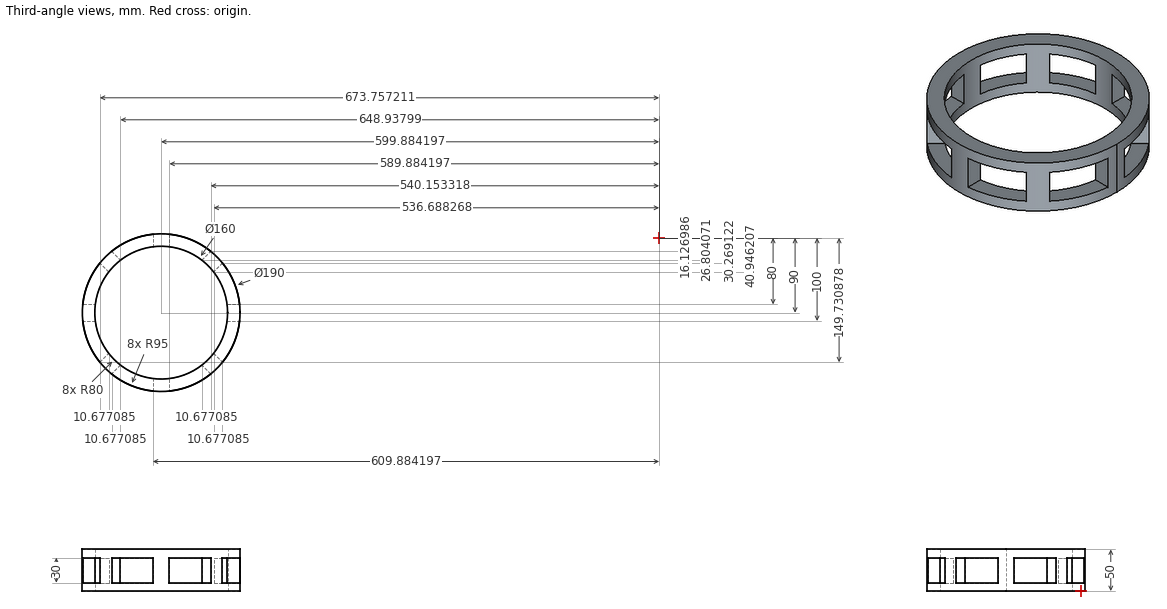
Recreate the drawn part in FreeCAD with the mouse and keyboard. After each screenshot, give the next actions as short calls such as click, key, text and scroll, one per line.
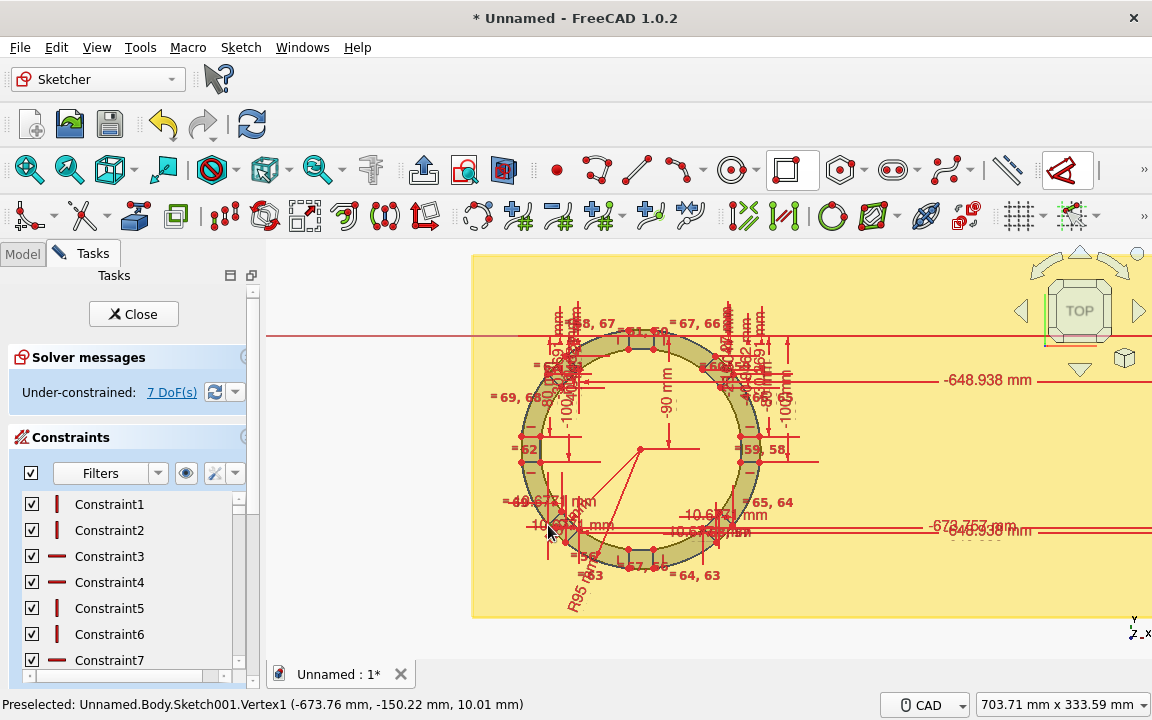
key(i)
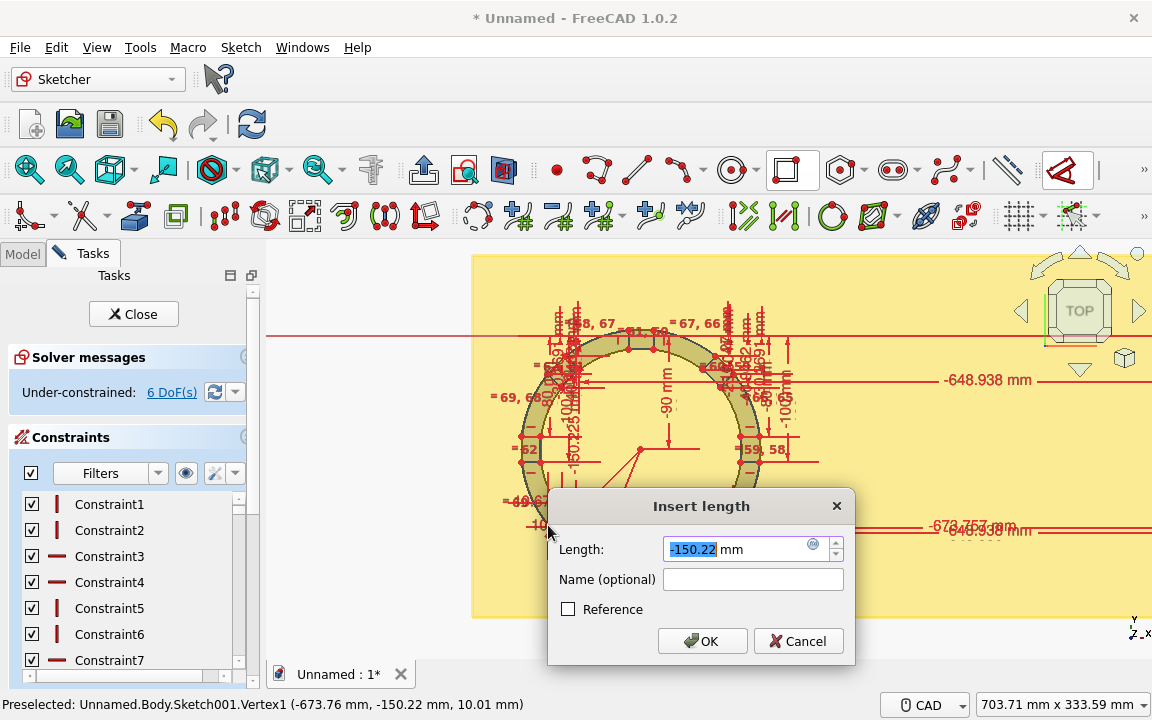
text(-149.730878)
key(Return)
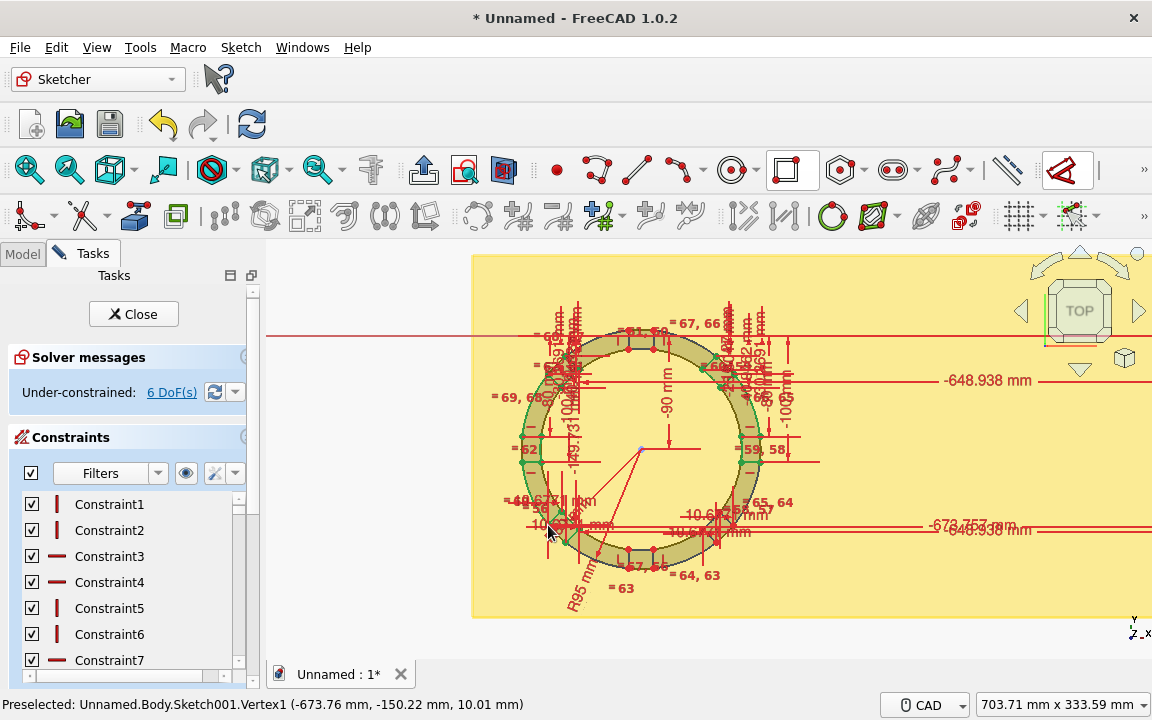
click(629, 568)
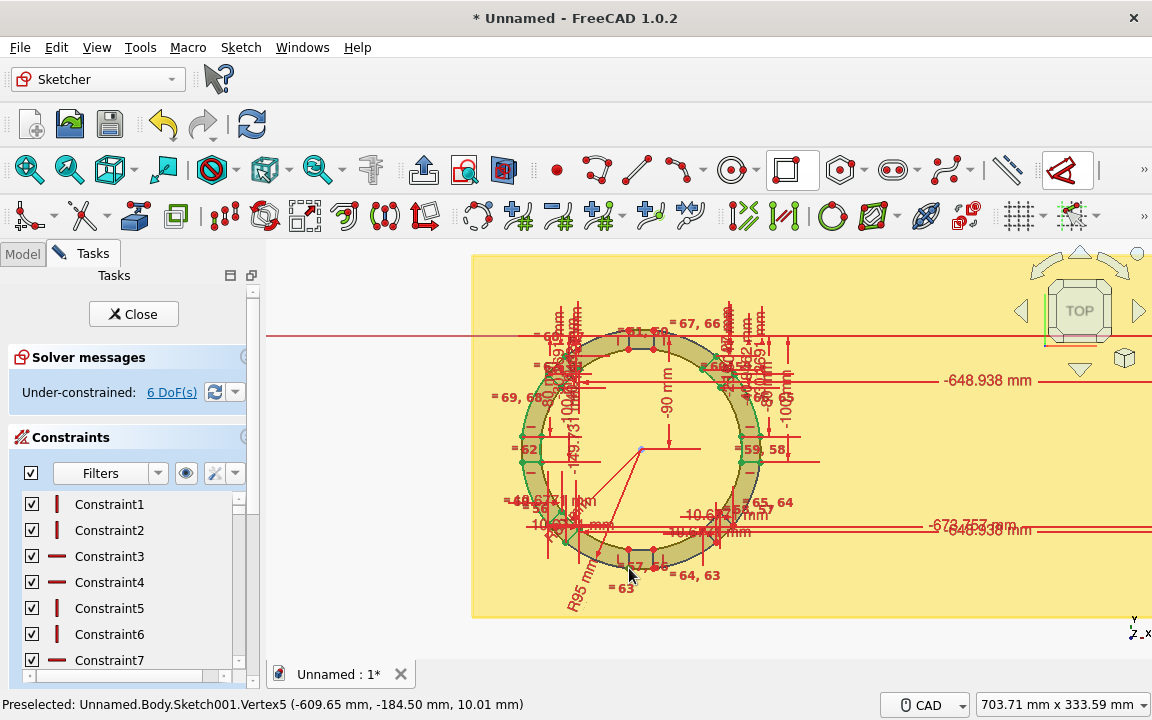
click(1088, 170)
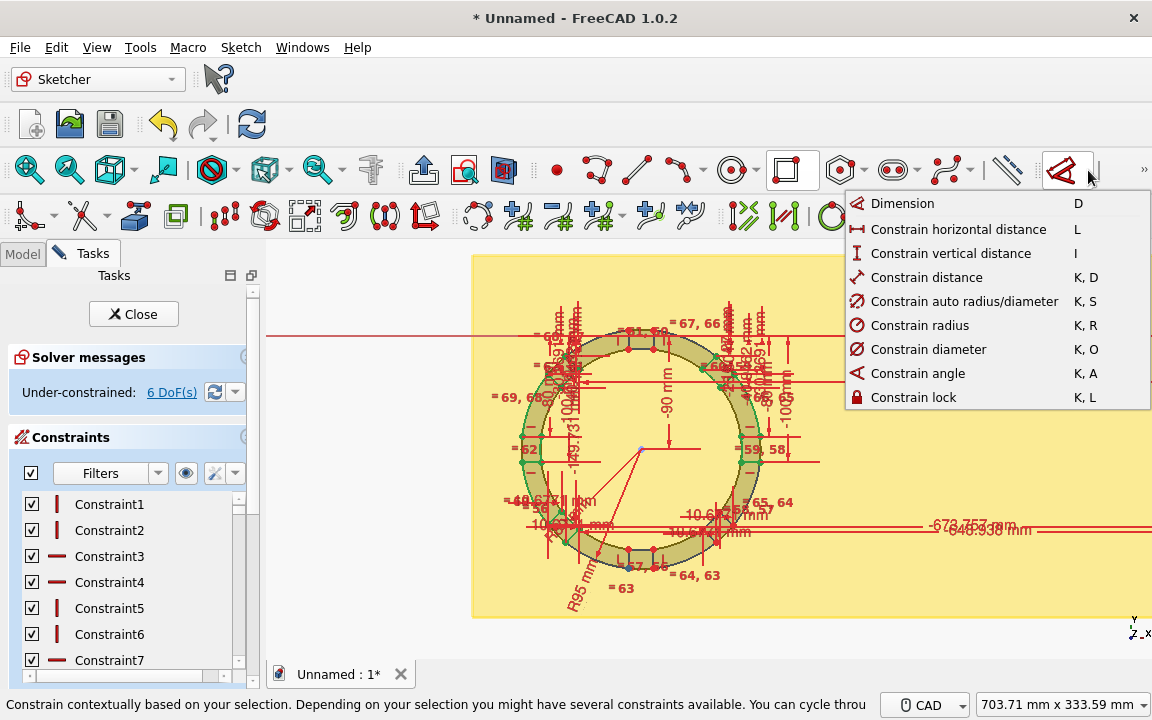
click(998, 229)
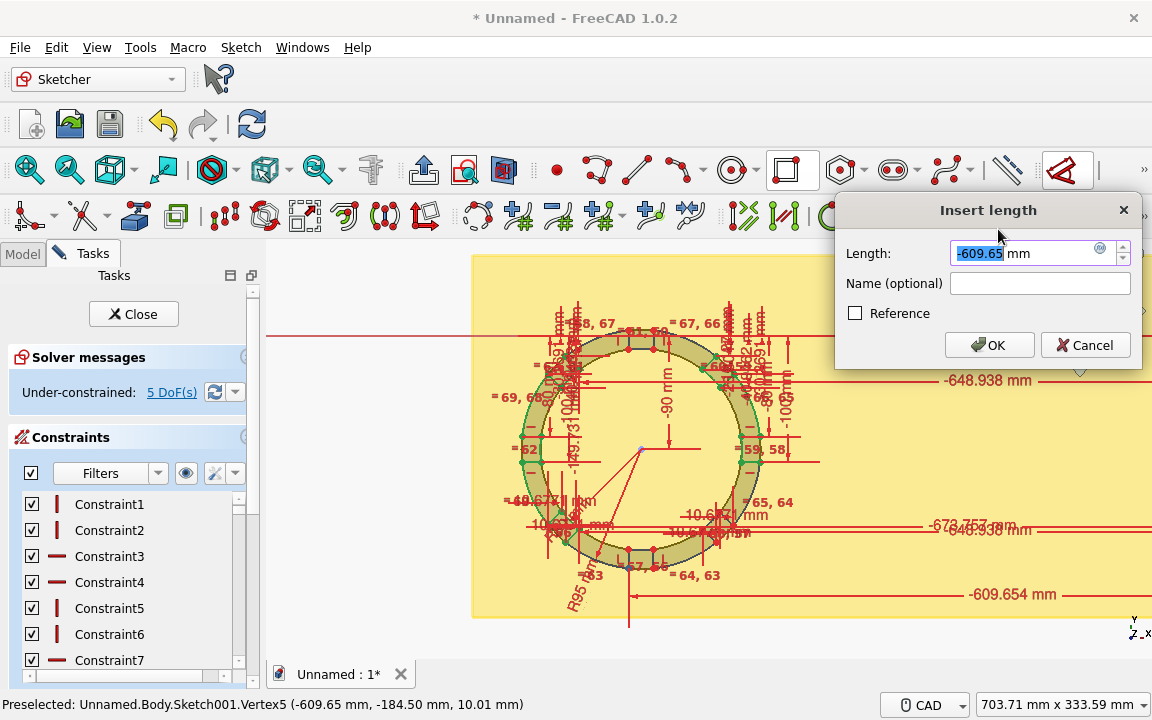
text(-609.884197)
key(Return)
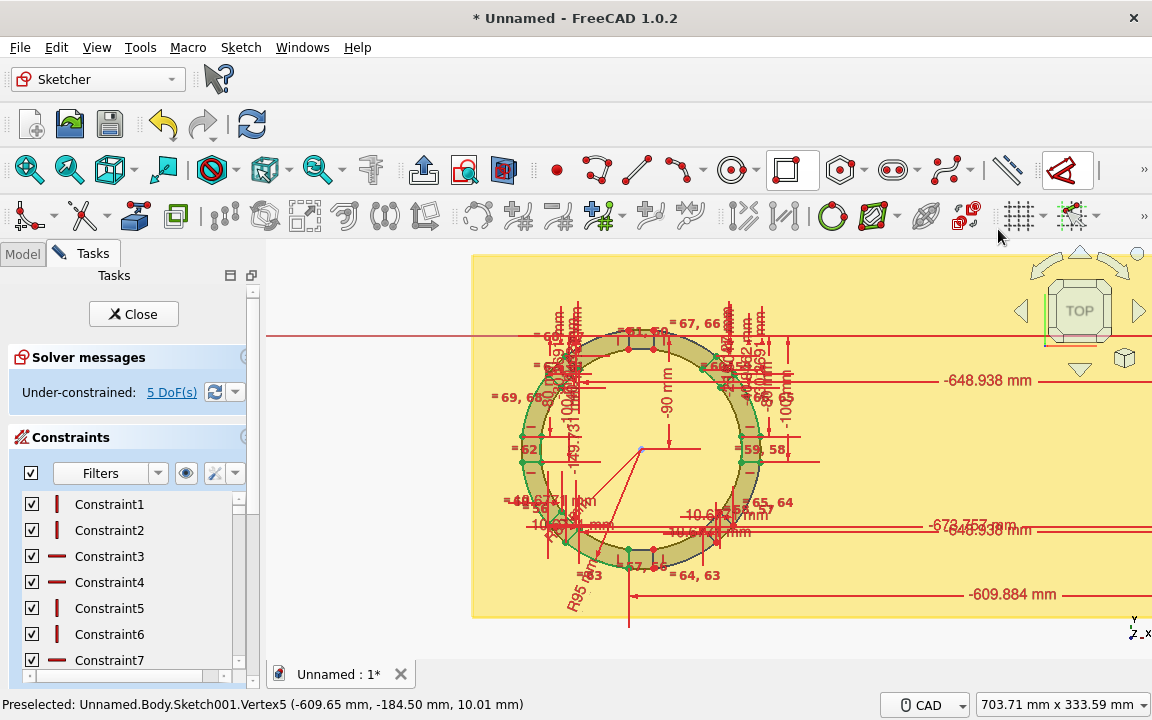
click(653, 549)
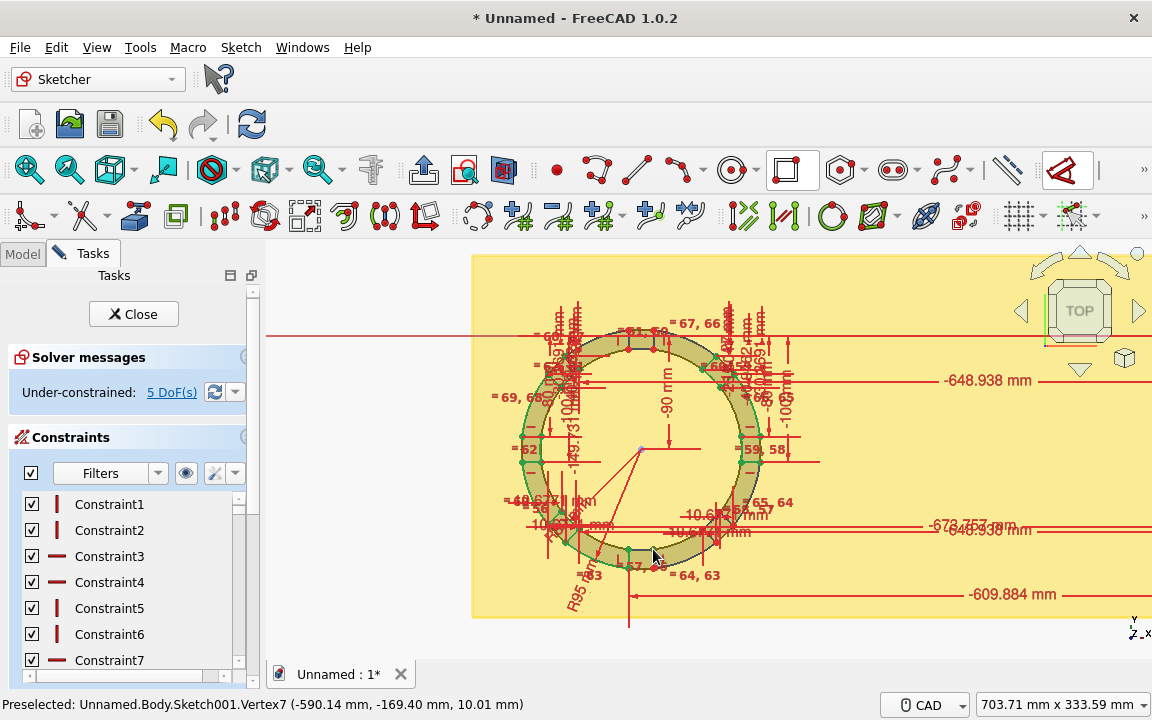
key(l)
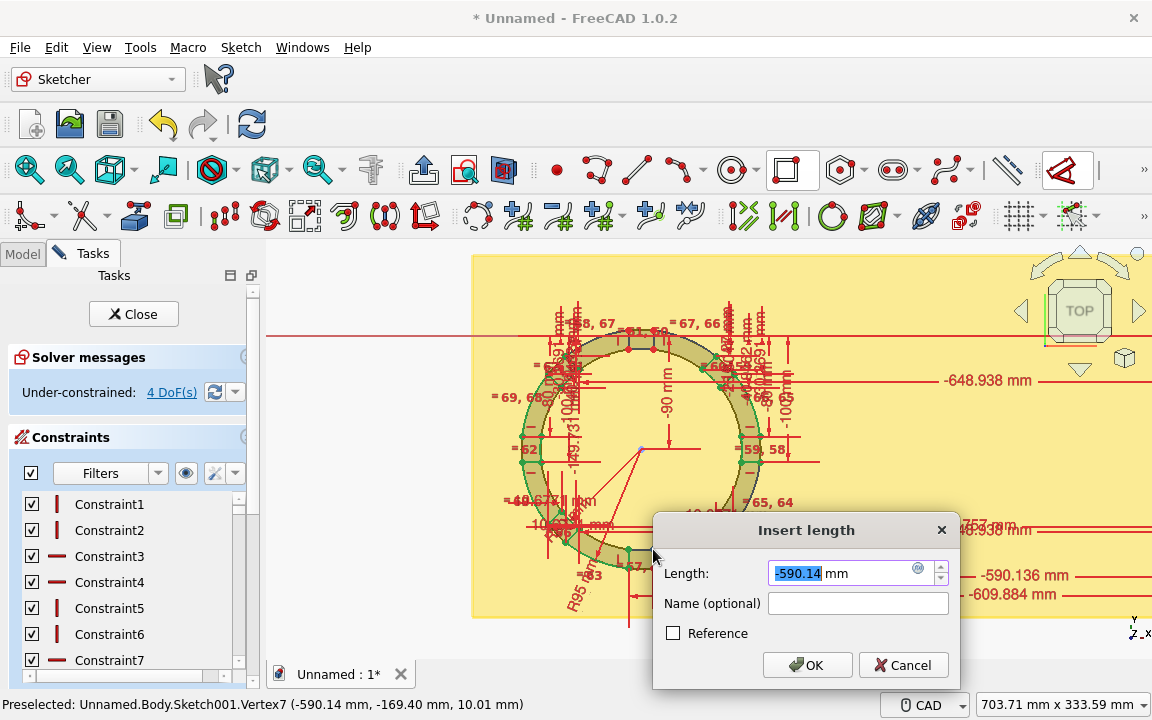
text(-589.884197)
key(Return)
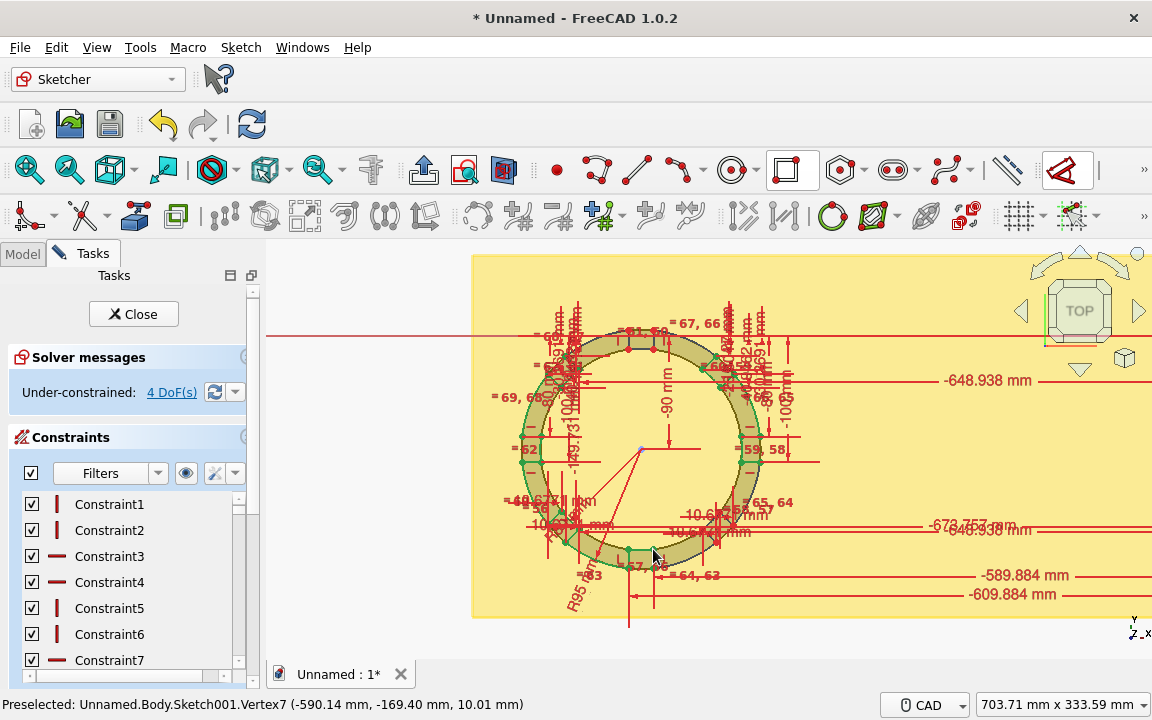
click(716, 542)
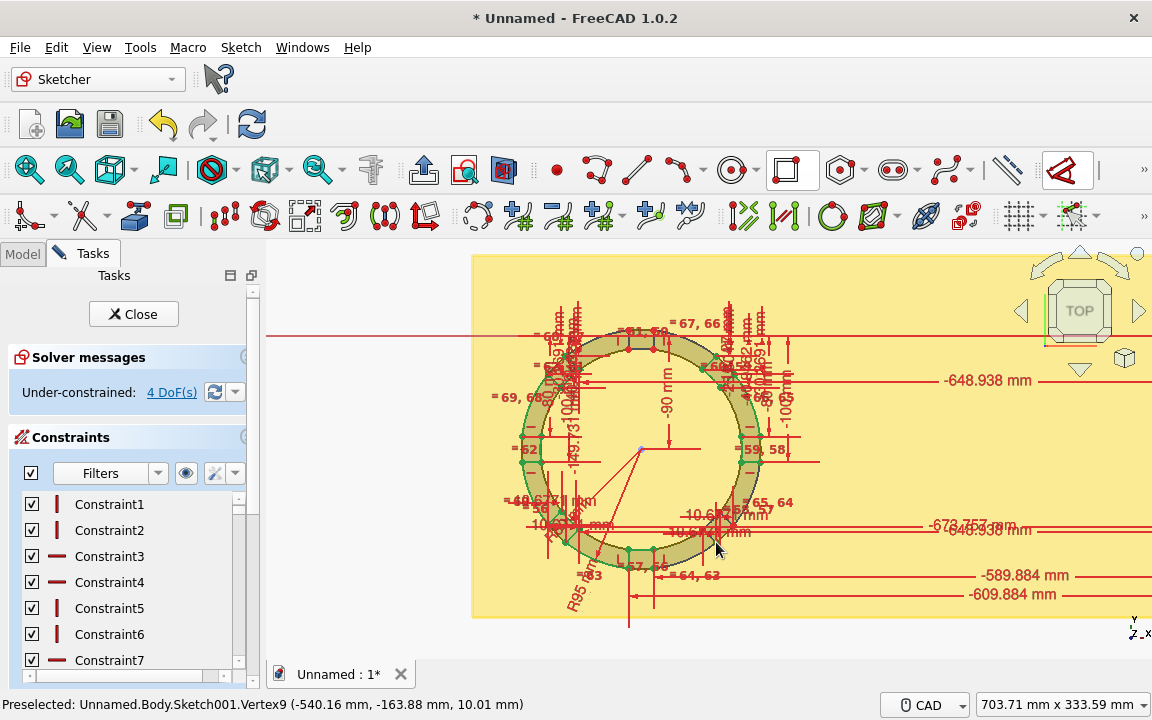
key(l)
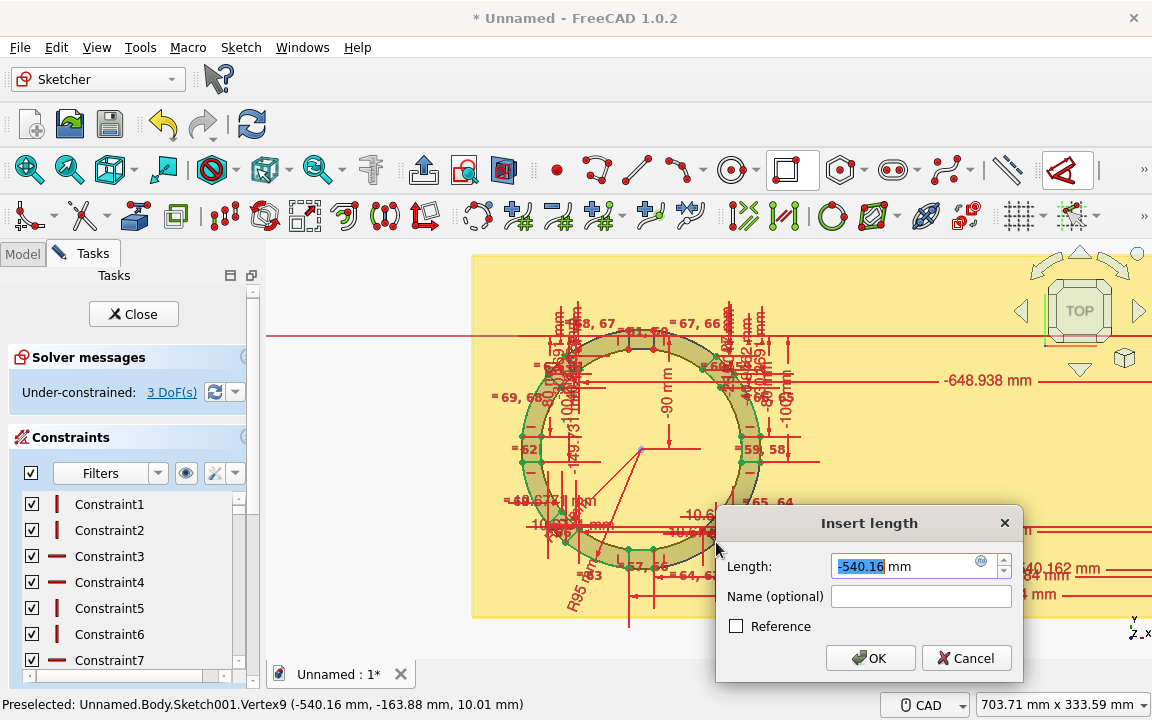
text(-540.153318)
key(Return)